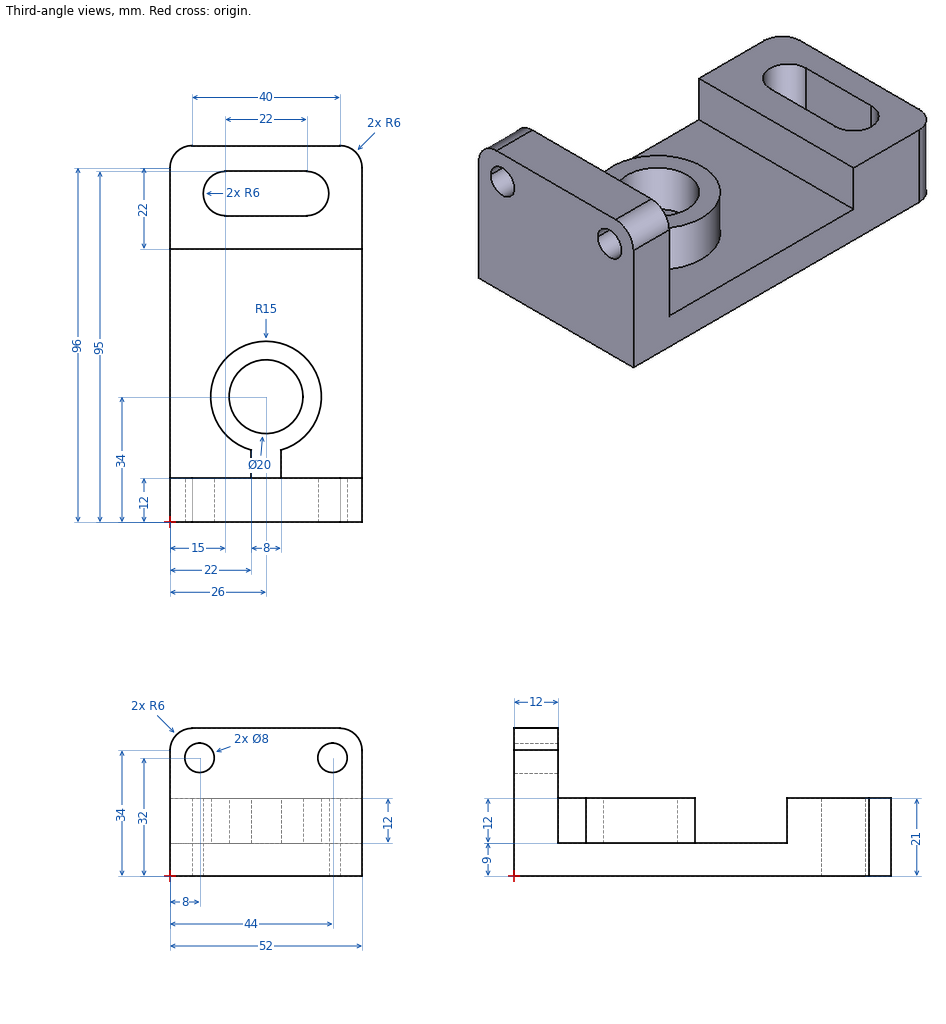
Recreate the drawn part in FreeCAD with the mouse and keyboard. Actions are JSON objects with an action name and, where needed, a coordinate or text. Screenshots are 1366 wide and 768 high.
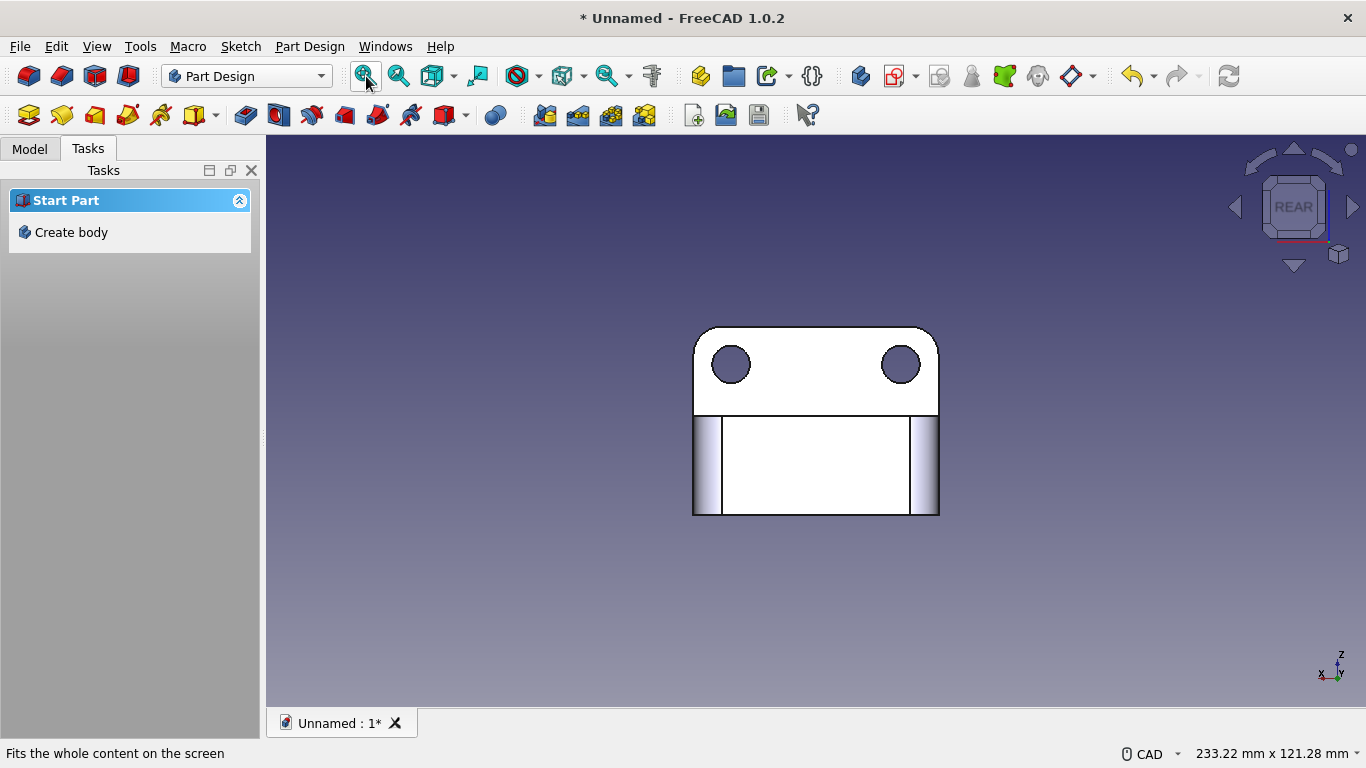
{"action": "key", "text": "0"}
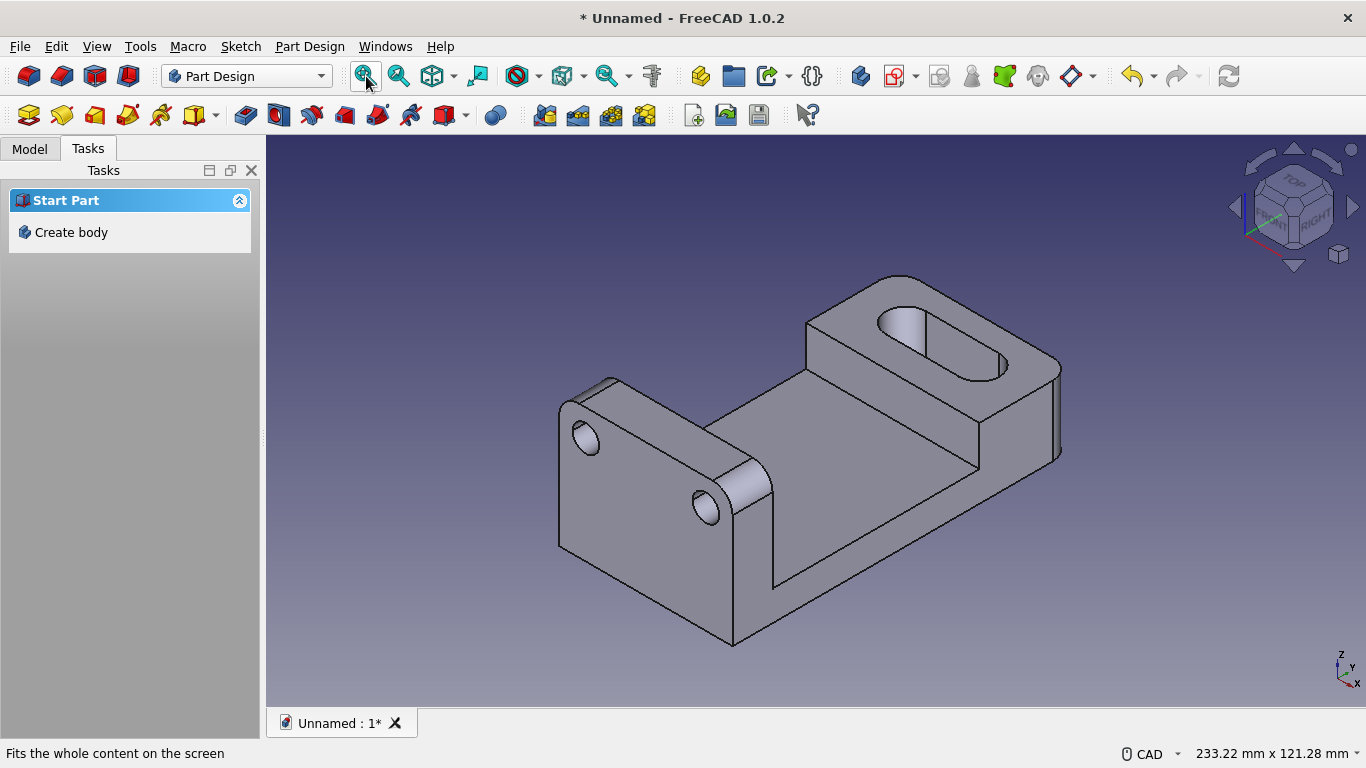
{"action": "left_click", "coordinate": [789, 478]}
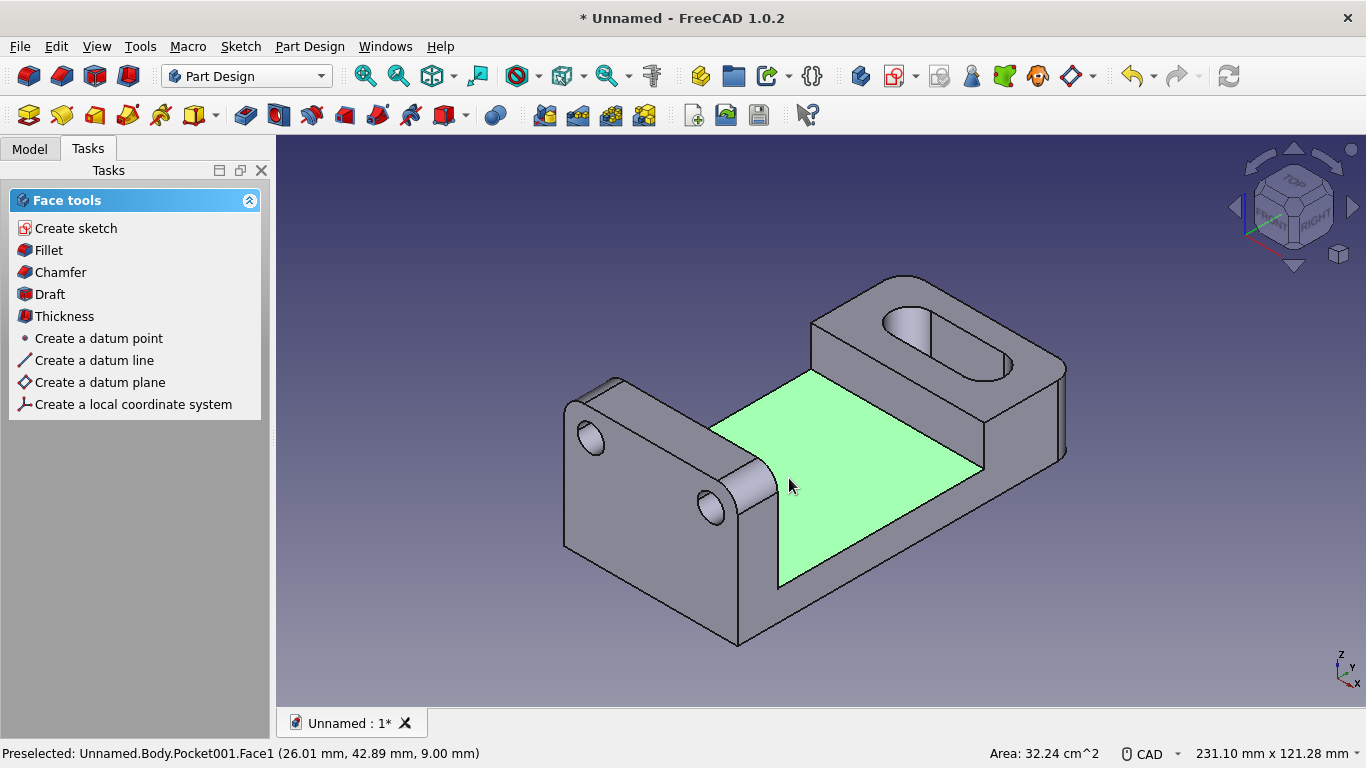
{"action": "left_click", "coordinate": [894, 76]}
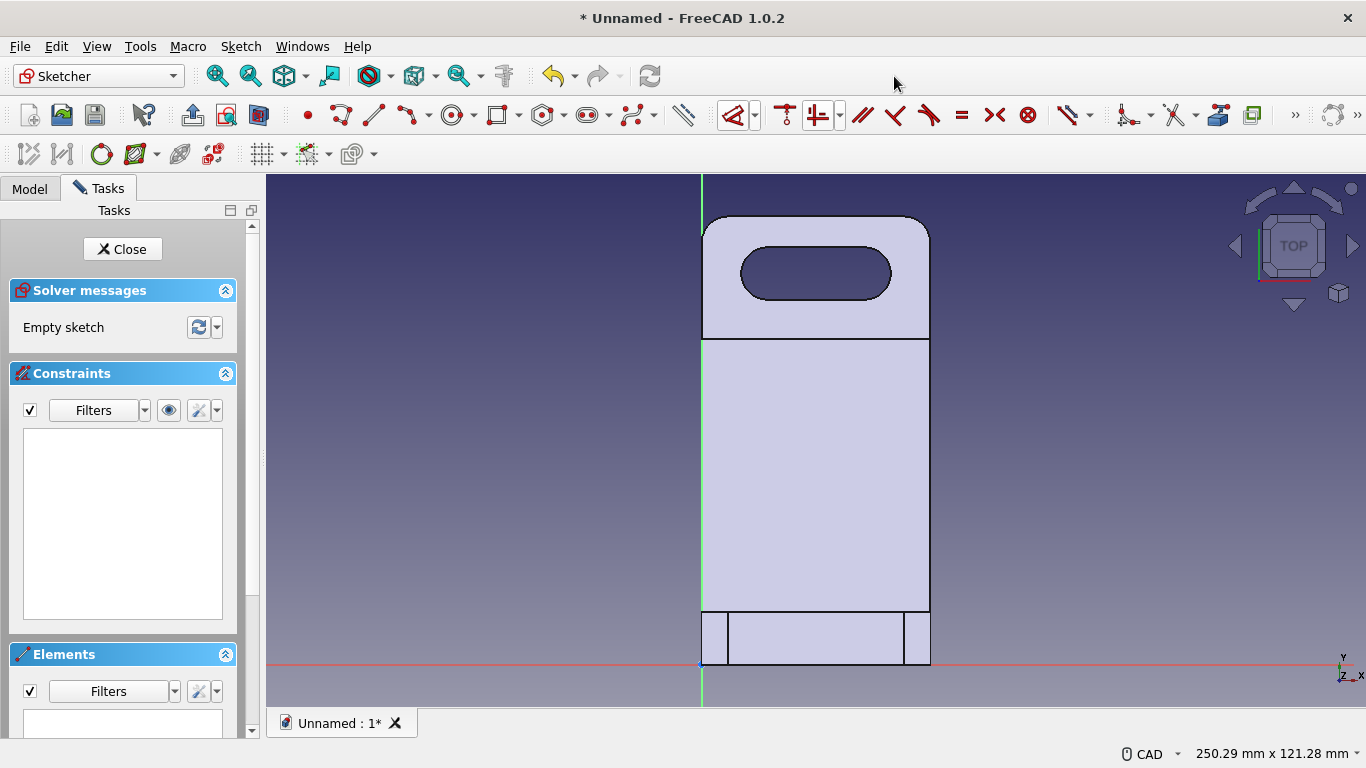
{"action": "scroll", "coordinate": [656, 202], "scroll_direction": "down", "scroll_amount": 1}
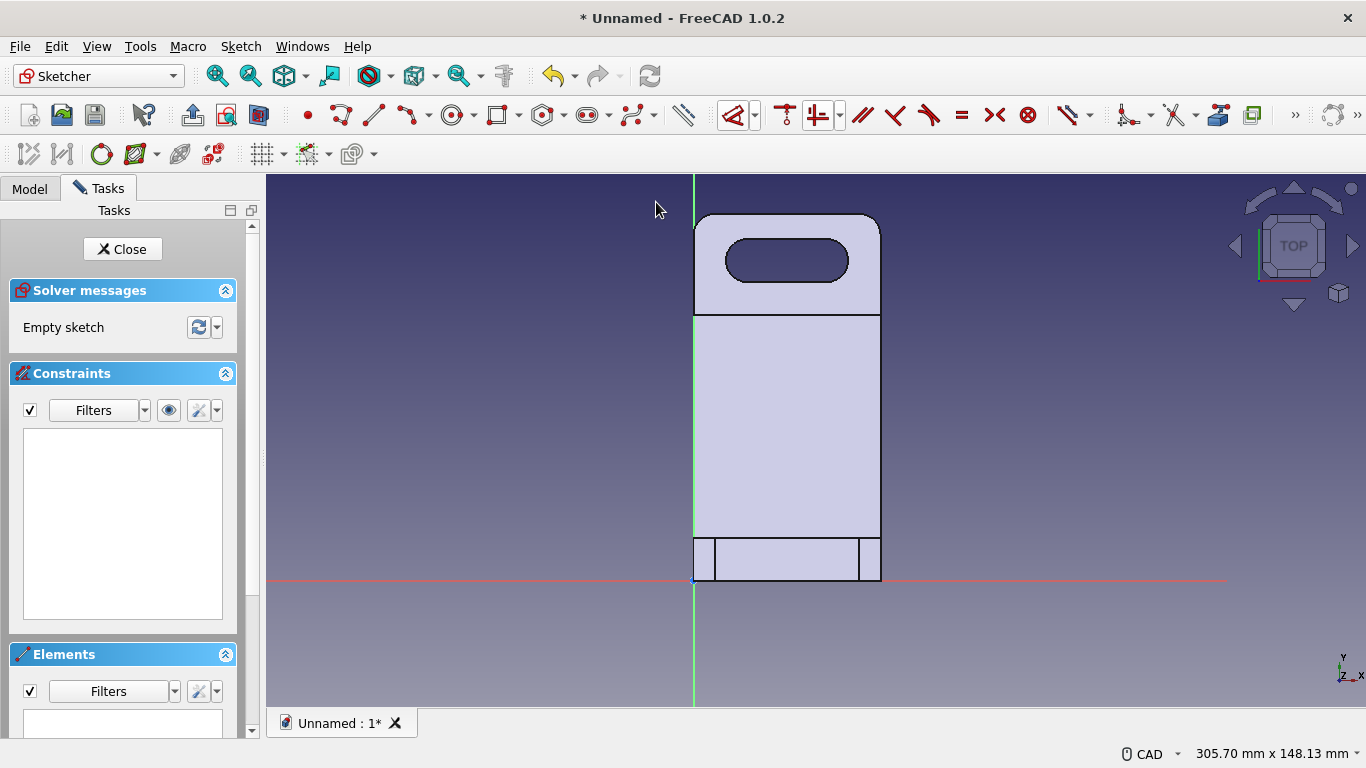
{"action": "scroll", "coordinate": [747, 556], "scroll_direction": "up", "scroll_amount": 3}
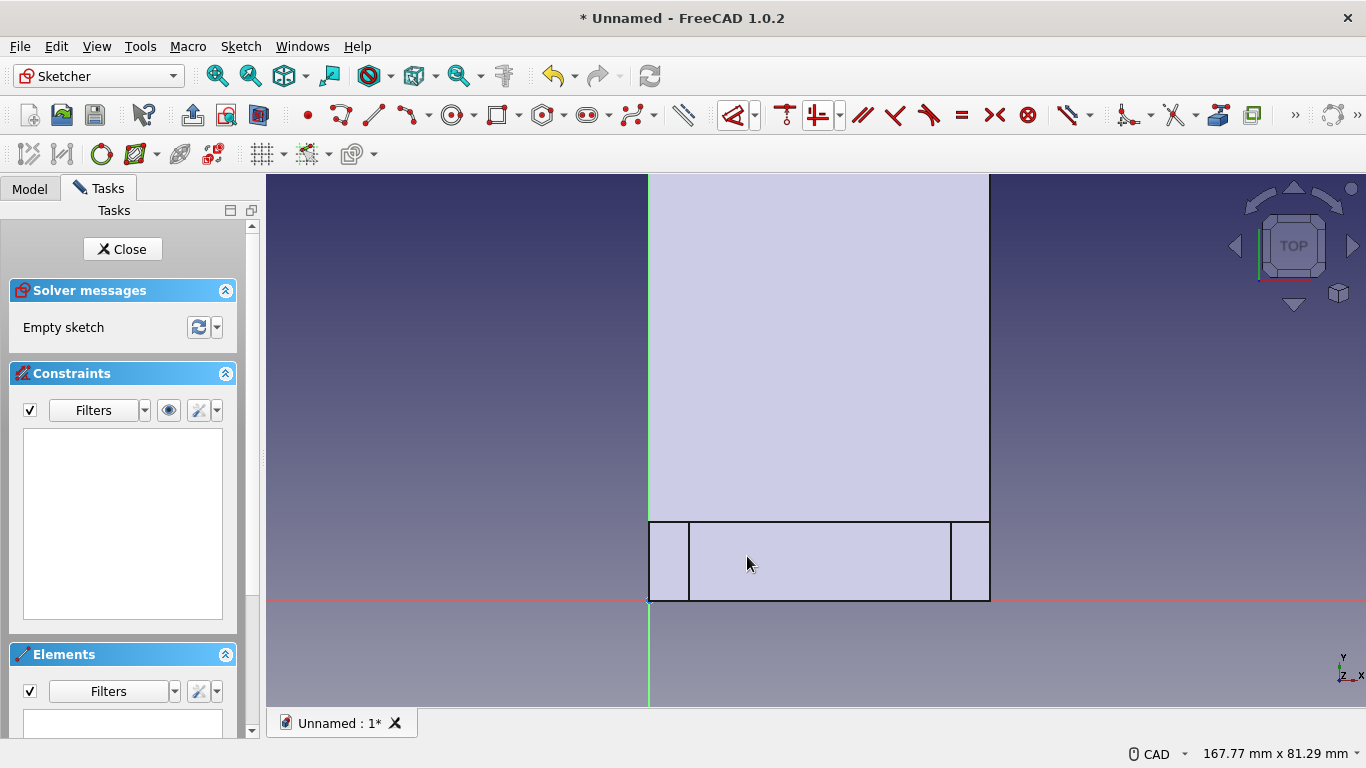
{"action": "left_click", "coordinate": [341, 116]}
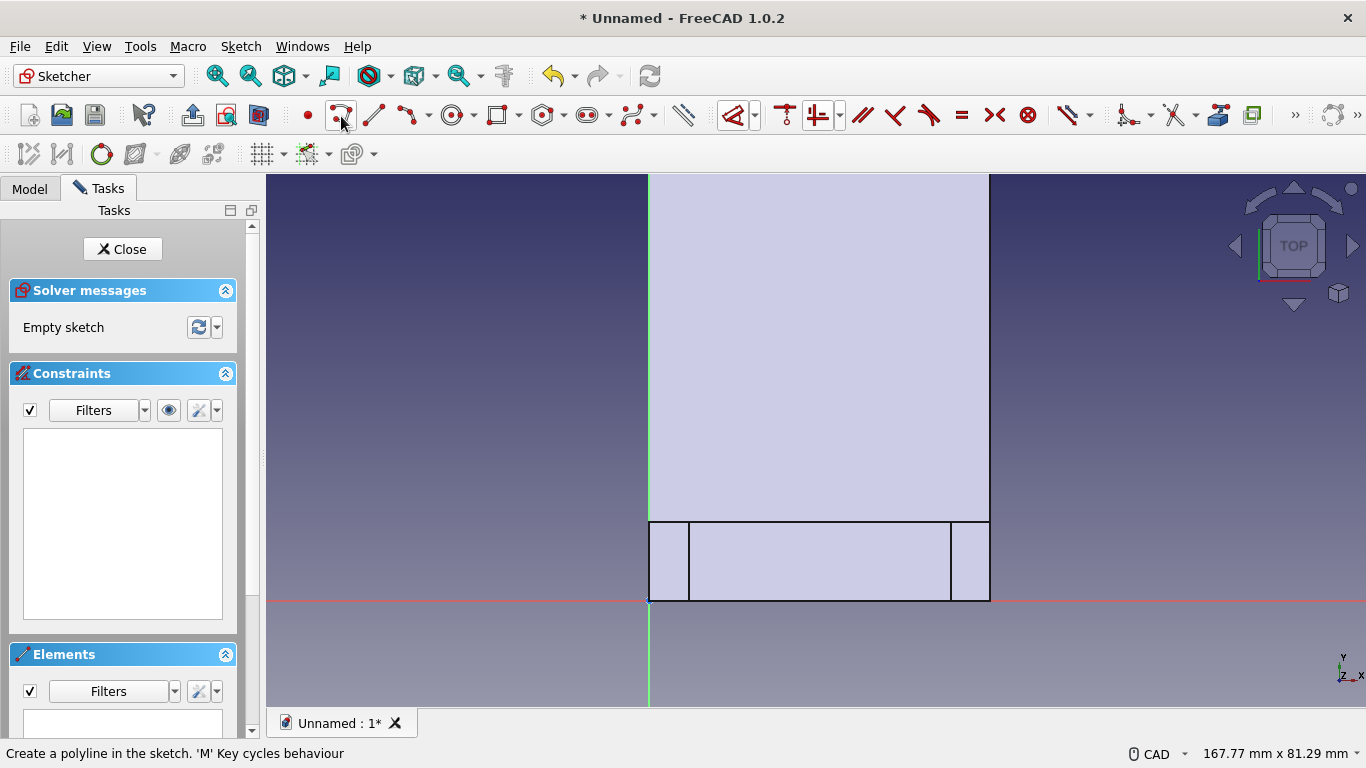
{"action": "left_click", "coordinate": [793, 472]}
{"action": "left_click", "coordinate": [793, 522]}
{"action": "left_click", "coordinate": [846, 522]}
{"action": "left_click", "coordinate": [846, 472]}
{"action": "right_click", "coordinate": [846, 472]}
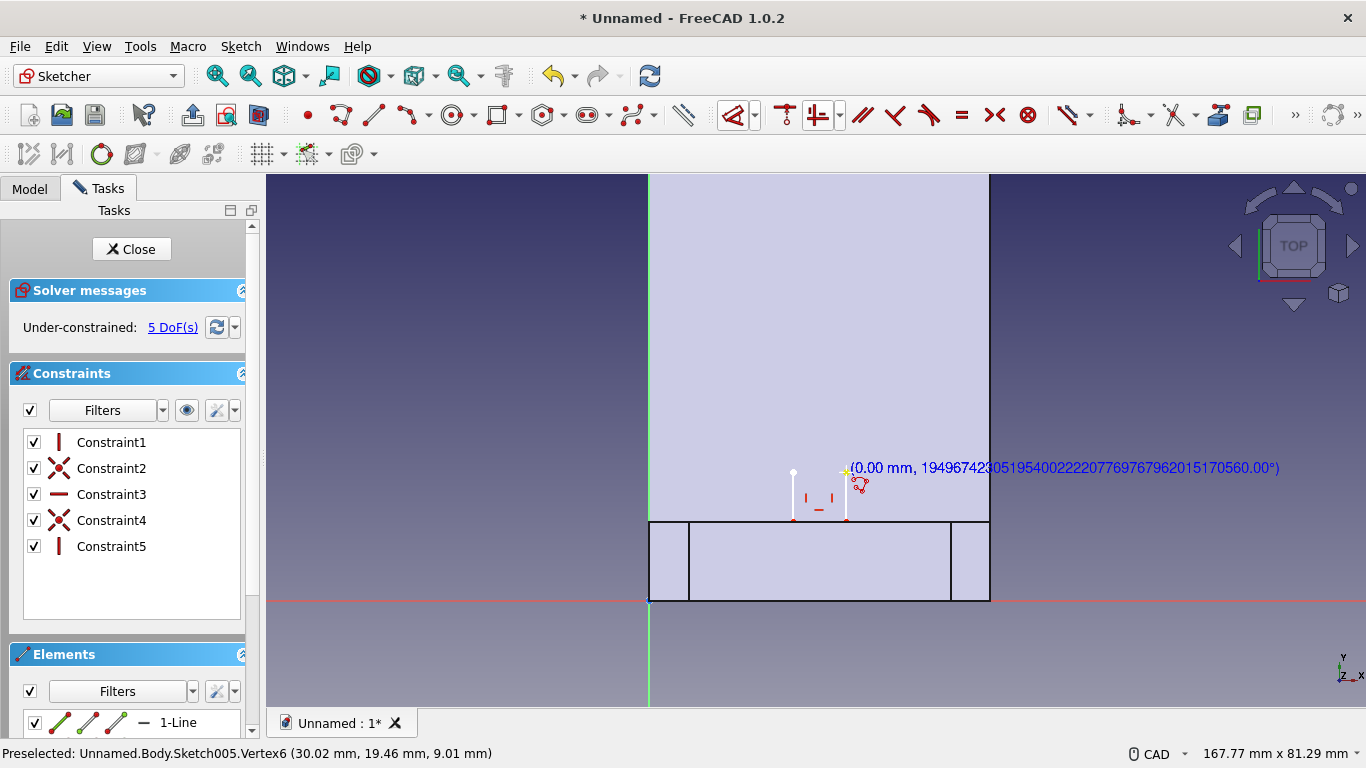
{"action": "left_click", "coordinate": [406, 116]}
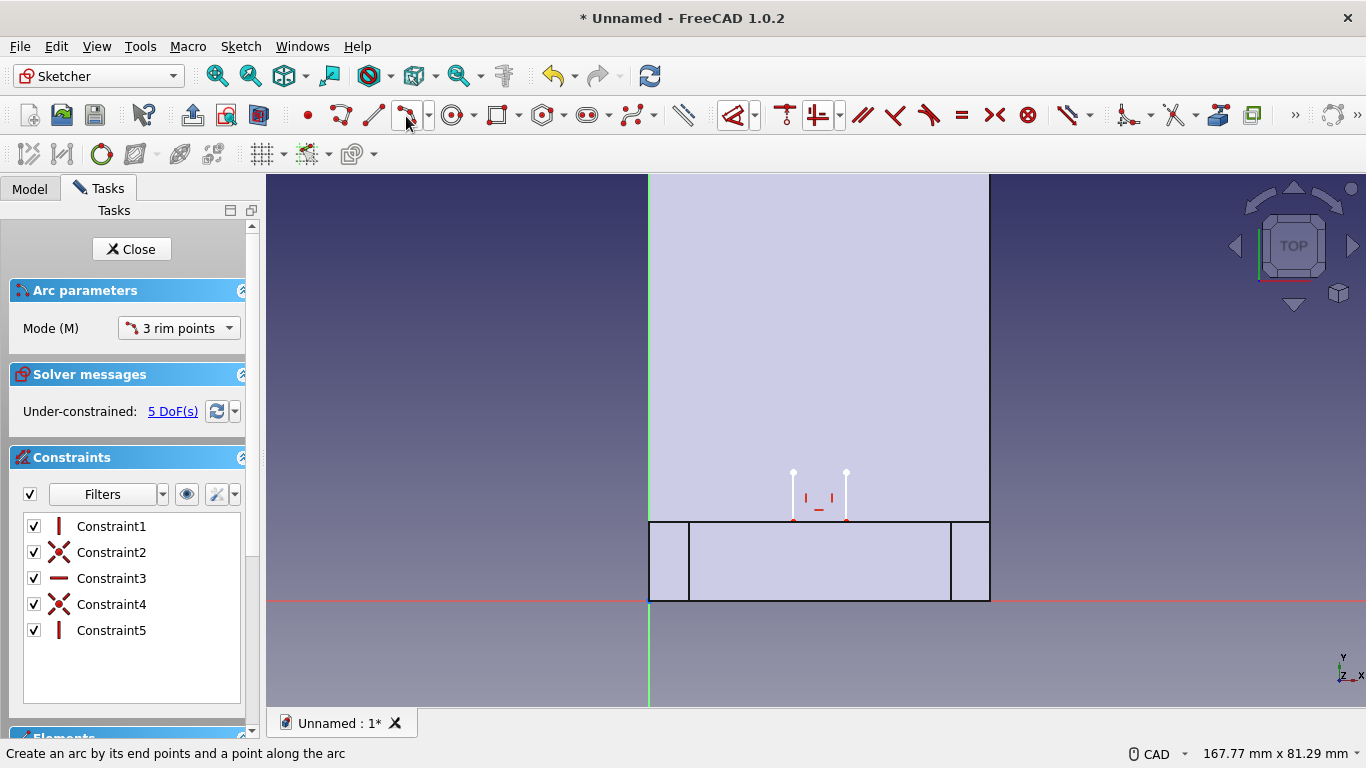
{"action": "left_click", "coordinate": [846, 473]}
{"action": "left_click", "coordinate": [793, 473]}
{"action": "left_click", "coordinate": [820, 279]}
{"action": "key", "text": "Escape"}